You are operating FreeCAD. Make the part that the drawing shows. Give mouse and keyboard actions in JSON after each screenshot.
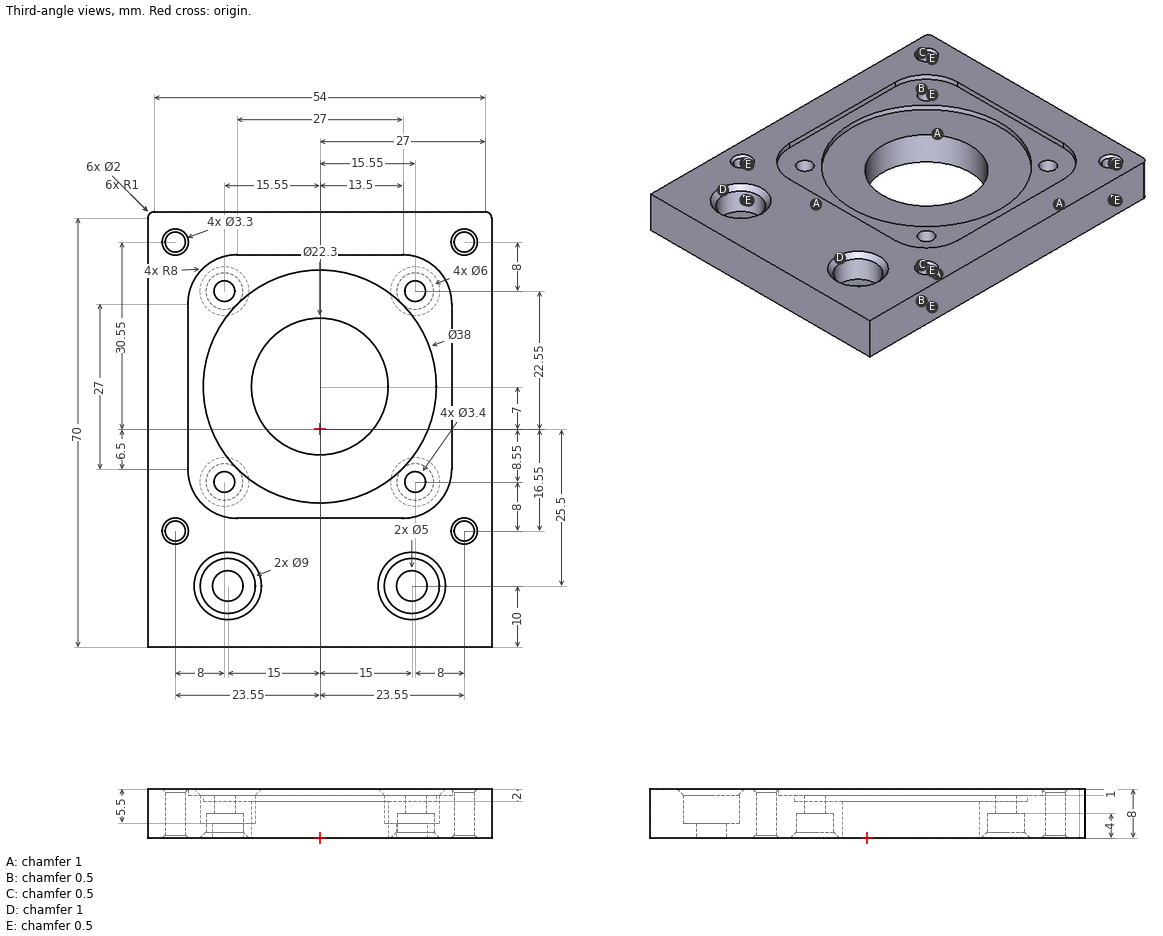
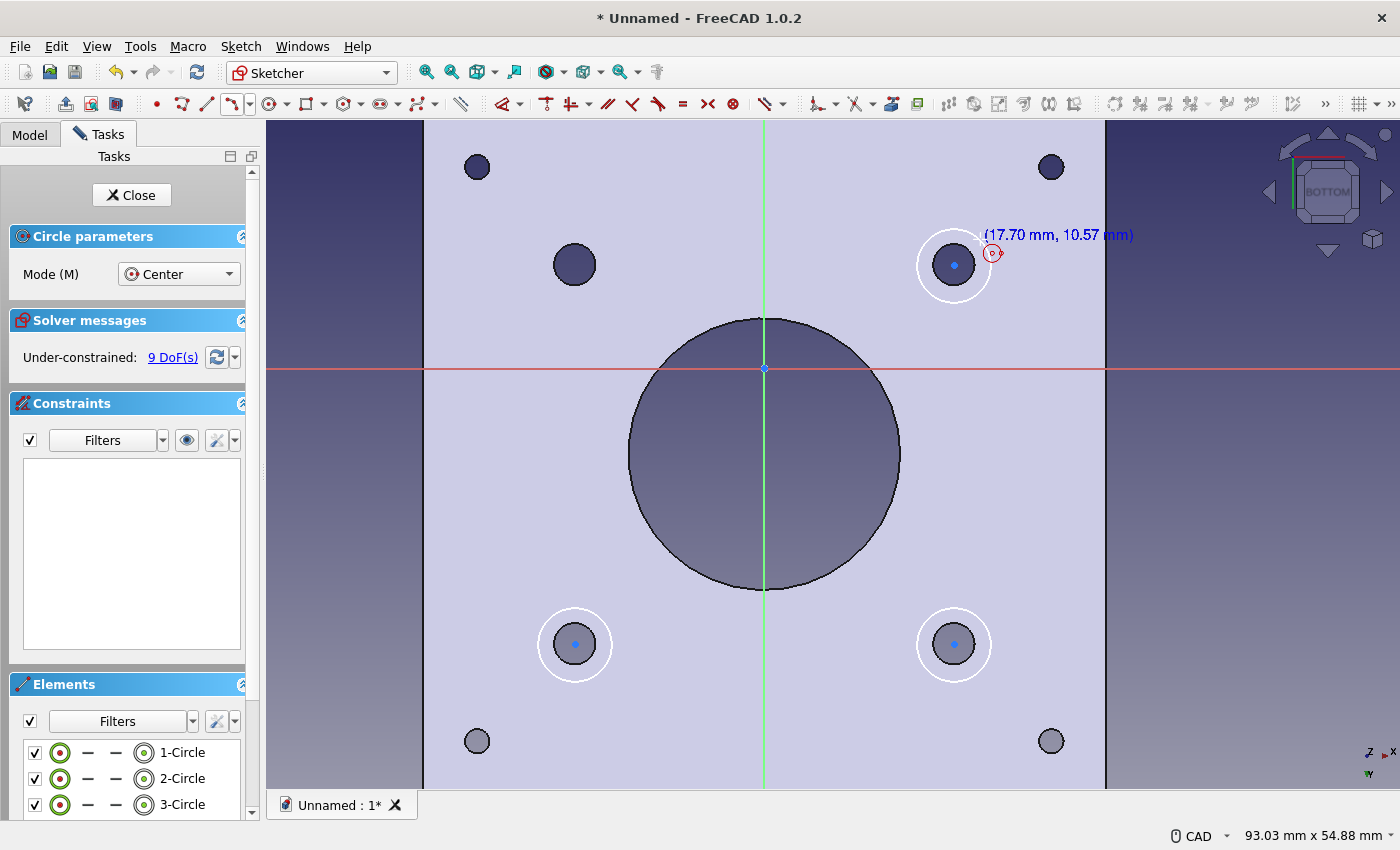
{"action": "left_click", "coordinate": [575, 265]}
{"action": "left_click", "coordinate": [601, 239]}
{"action": "key", "text": "Escape"}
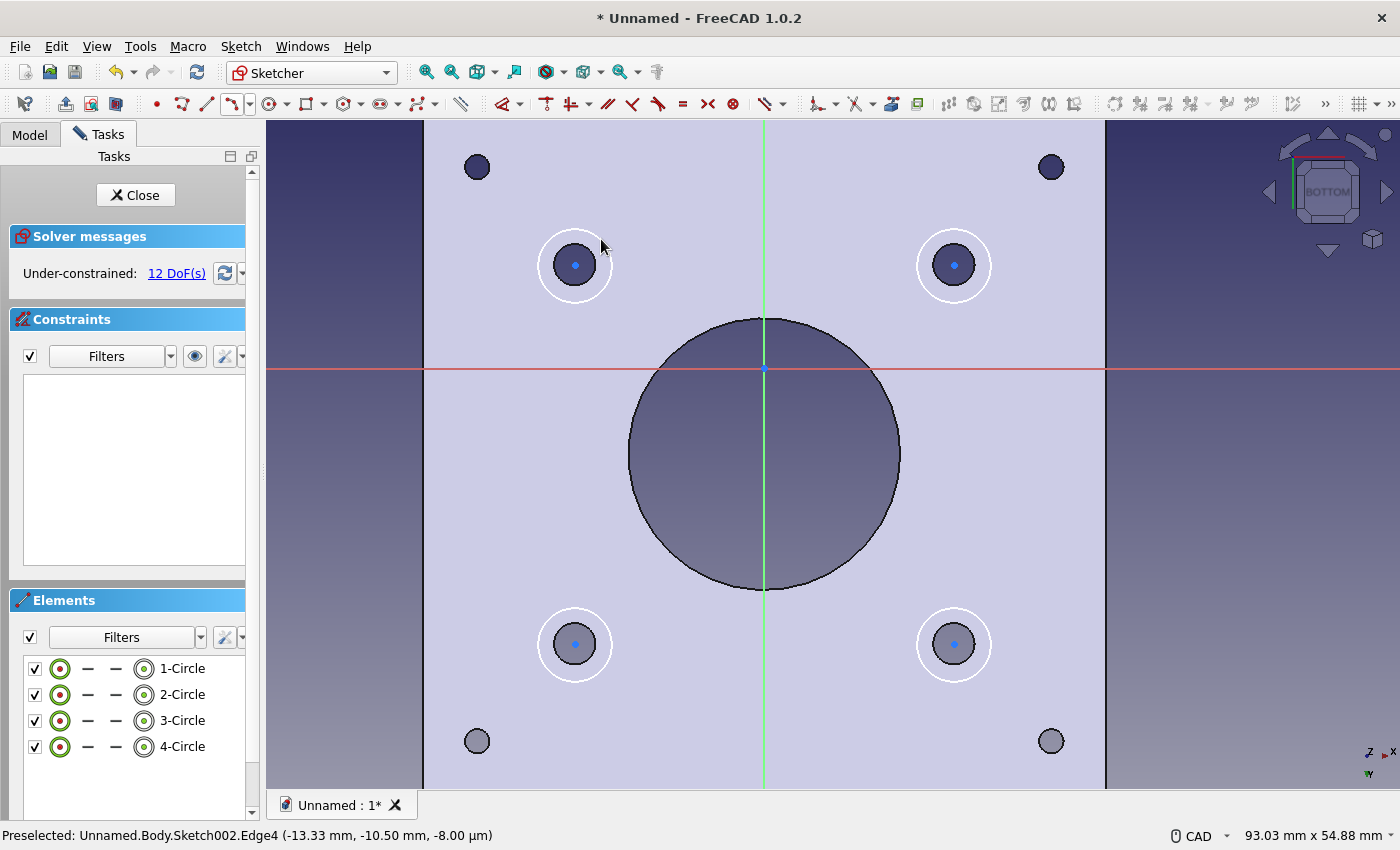
{"action": "left_click", "coordinate": [980, 619]}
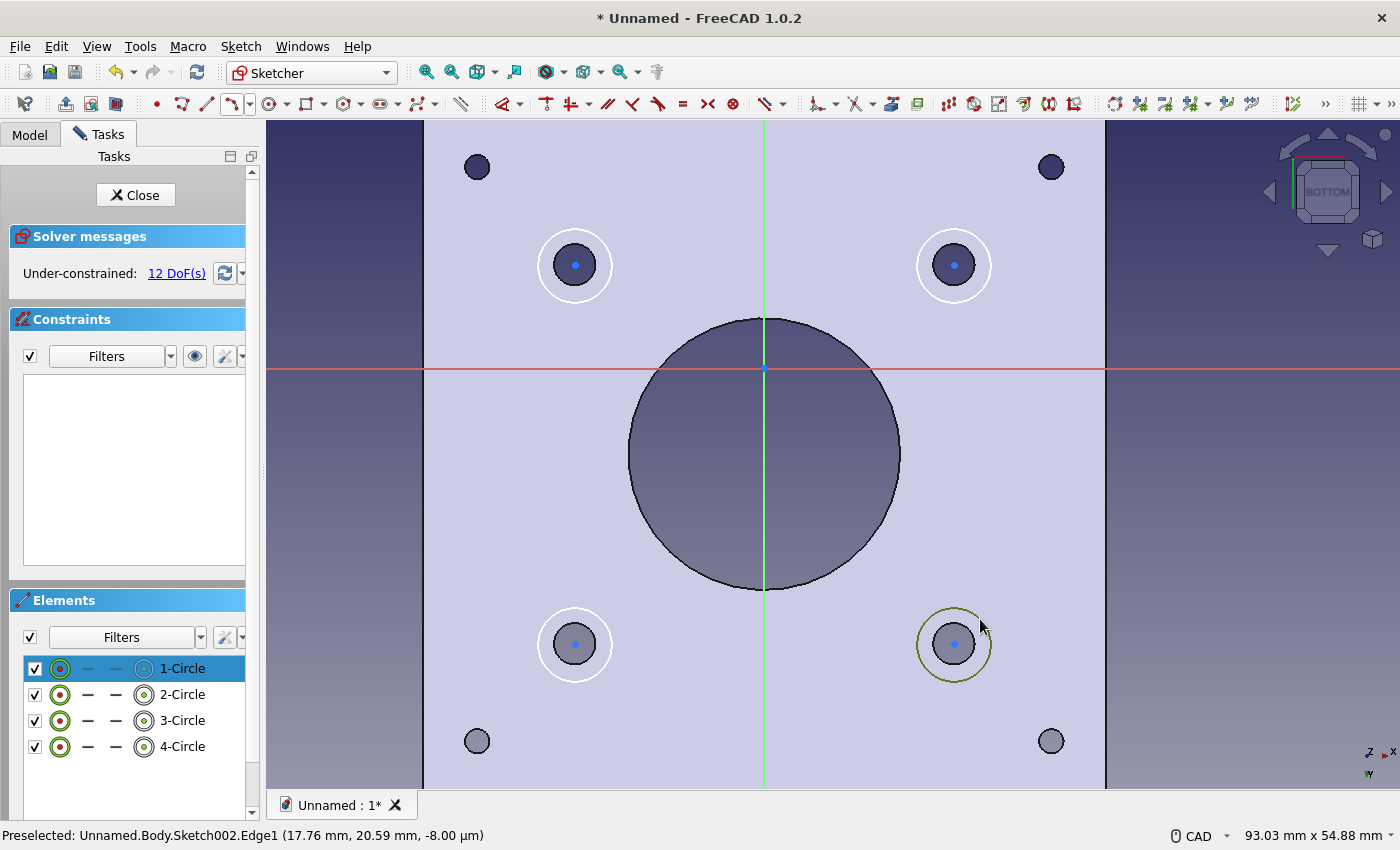
{"action": "left_click", "coordinate": [601, 619]}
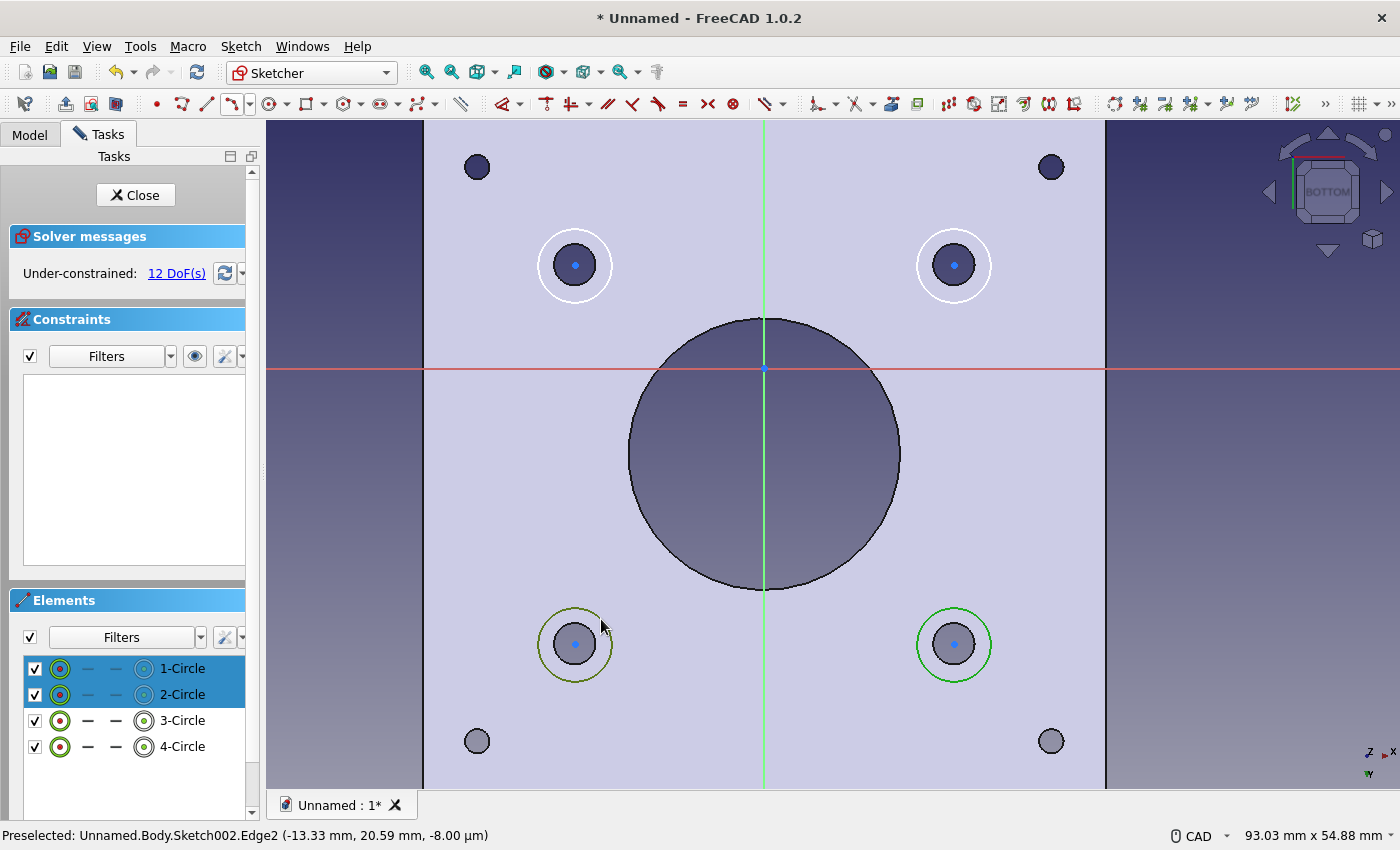
{"action": "left_click", "coordinate": [980, 240]}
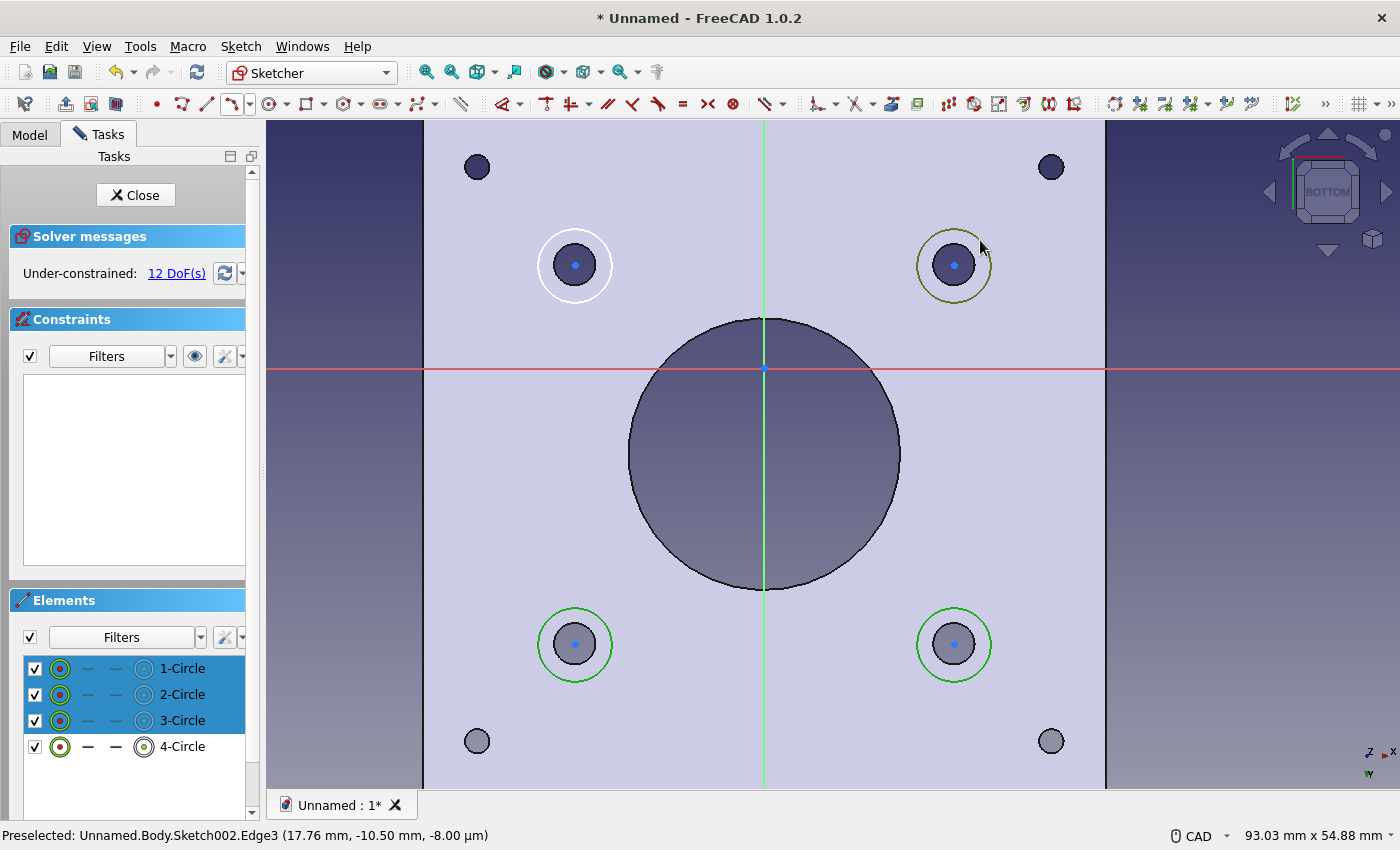
{"action": "left_click", "coordinate": [601, 240]}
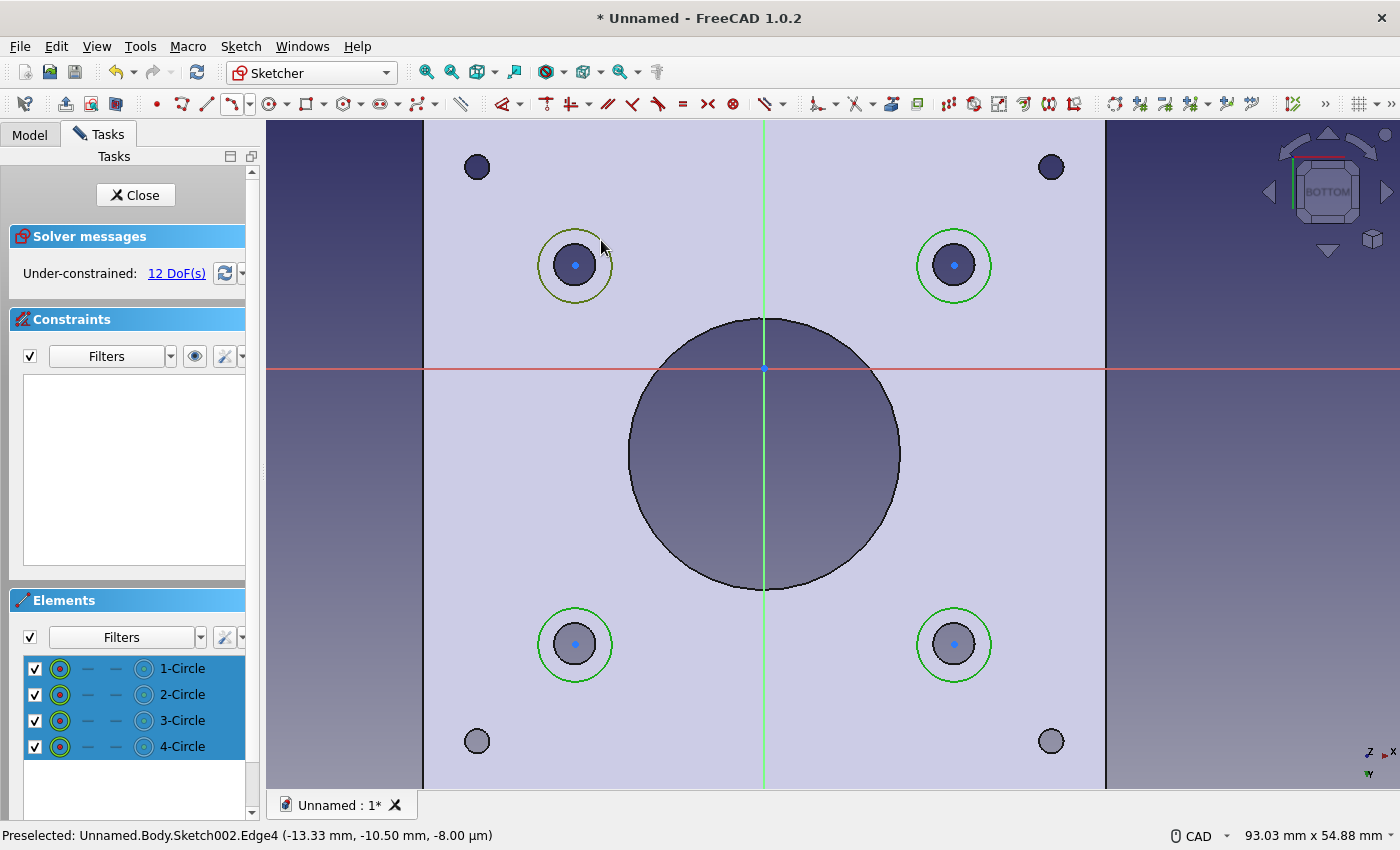
{"action": "key", "text": "e"}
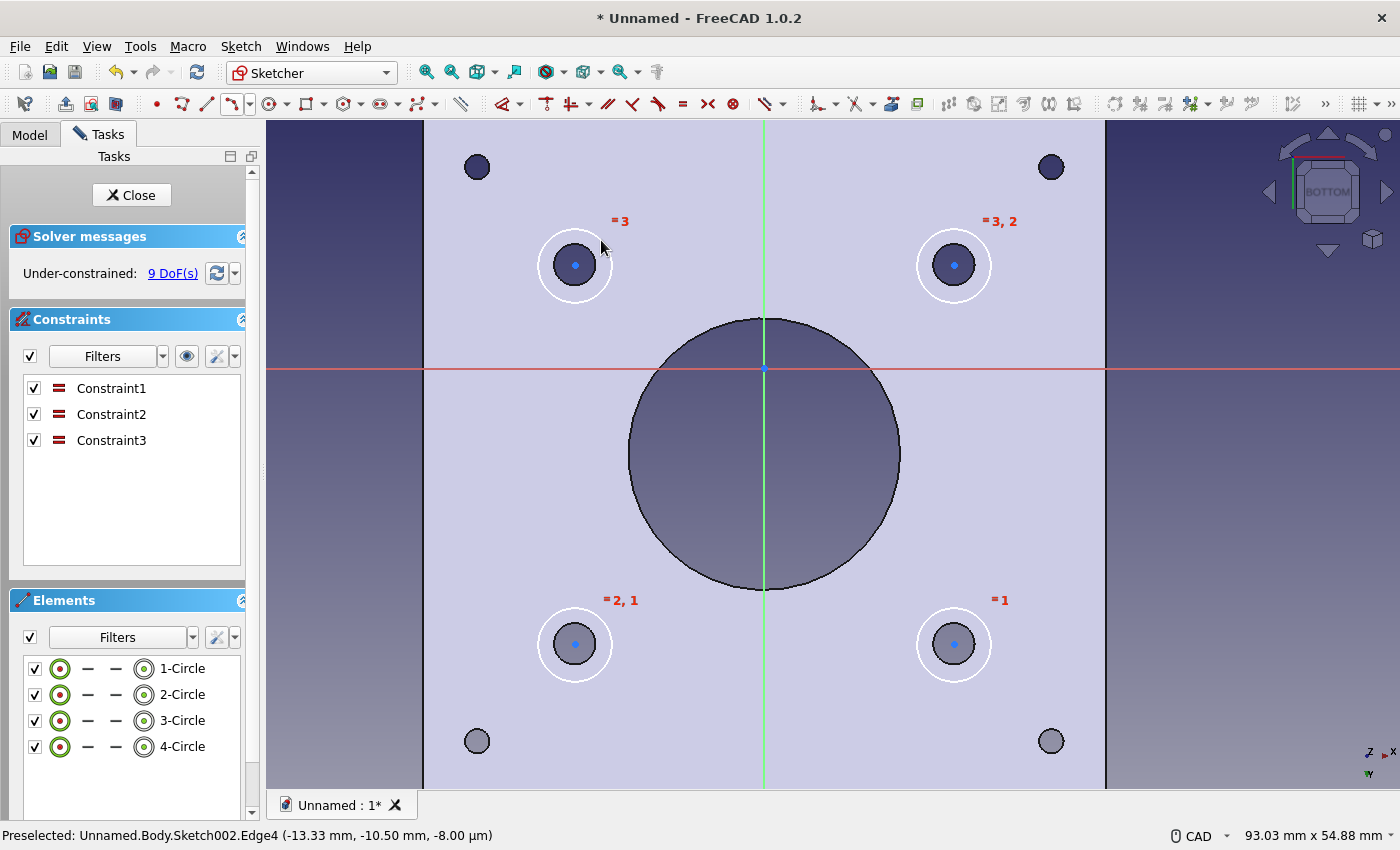
{"action": "left_click", "coordinate": [502, 104]}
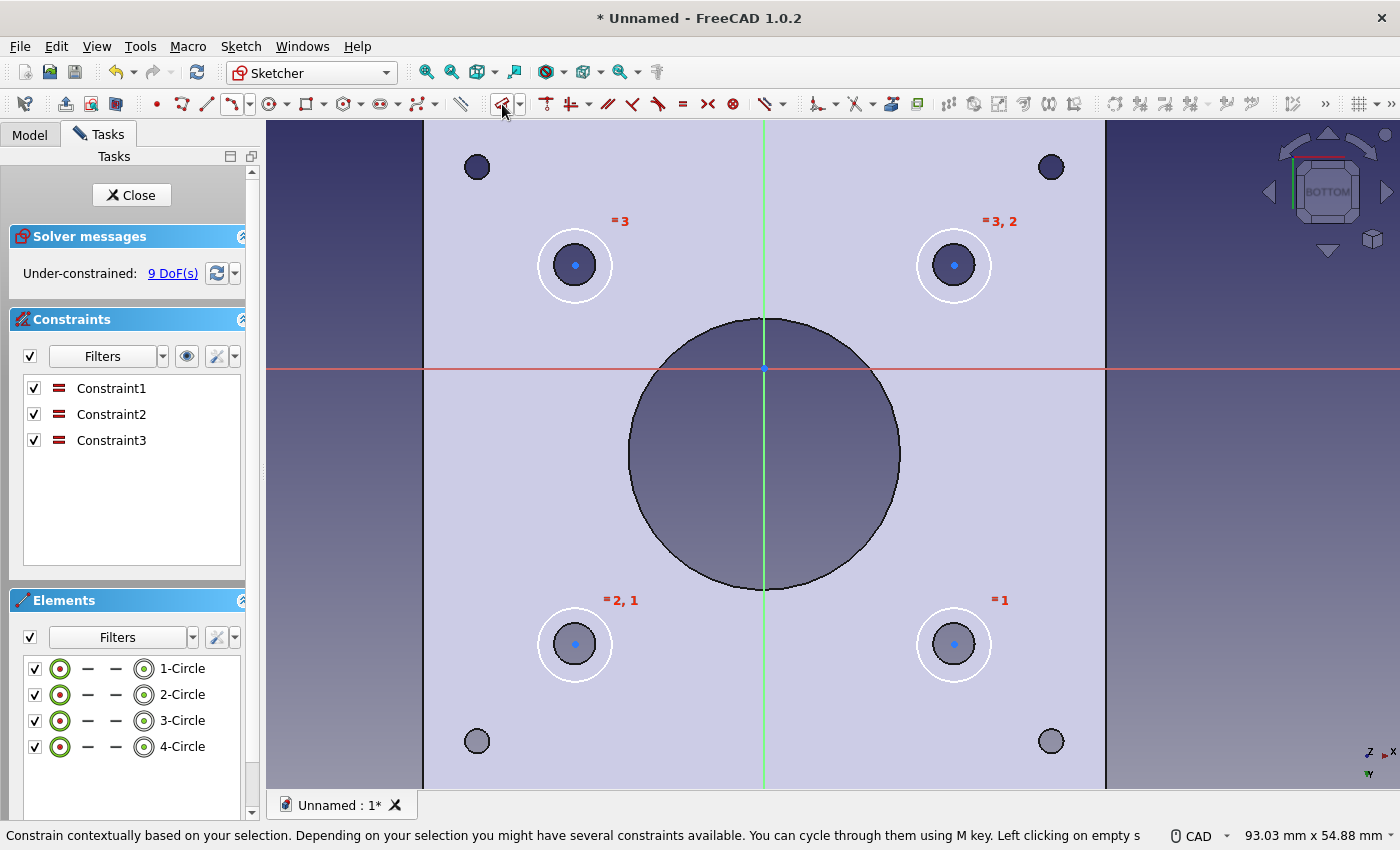
{"action": "left_click", "coordinate": [980, 619]}
{"action": "left_click", "coordinate": [1003, 596]}